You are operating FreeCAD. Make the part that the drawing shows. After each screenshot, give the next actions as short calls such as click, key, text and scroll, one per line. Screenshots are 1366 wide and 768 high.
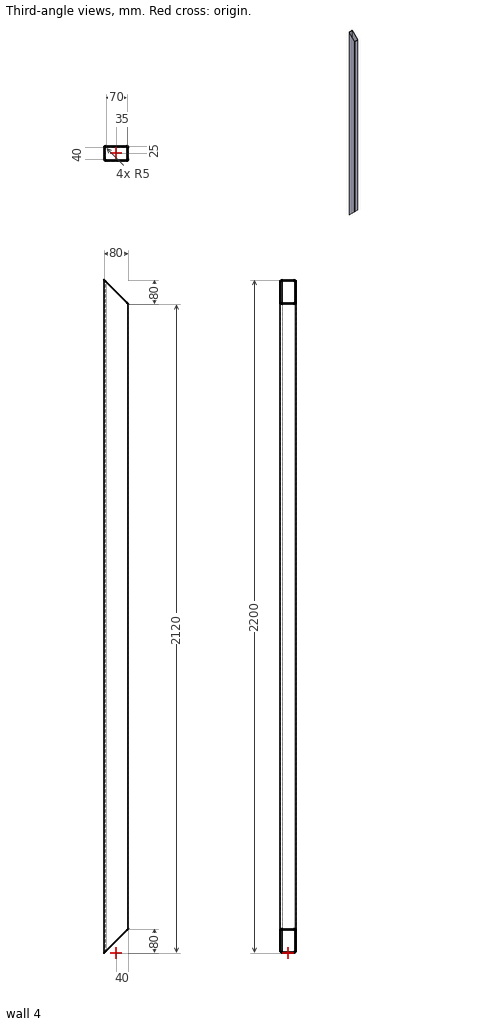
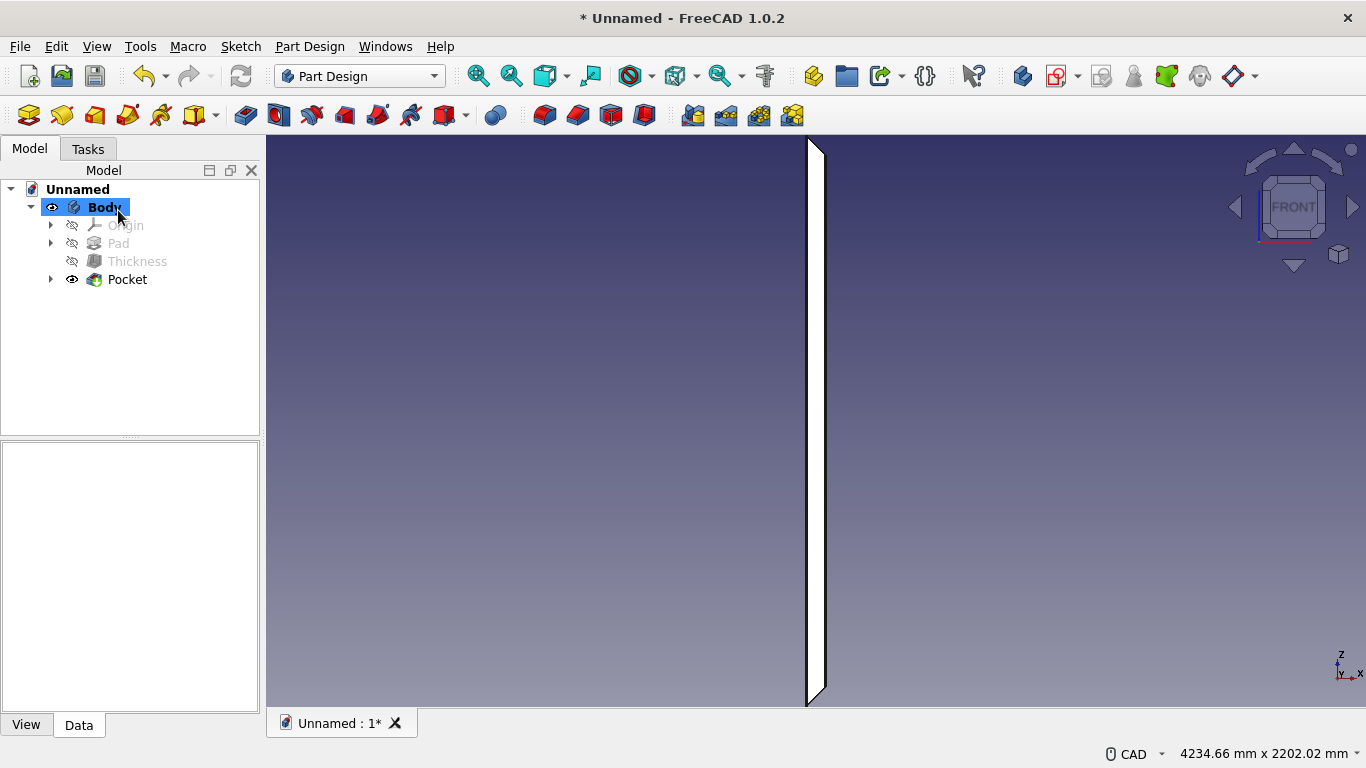
key(0)